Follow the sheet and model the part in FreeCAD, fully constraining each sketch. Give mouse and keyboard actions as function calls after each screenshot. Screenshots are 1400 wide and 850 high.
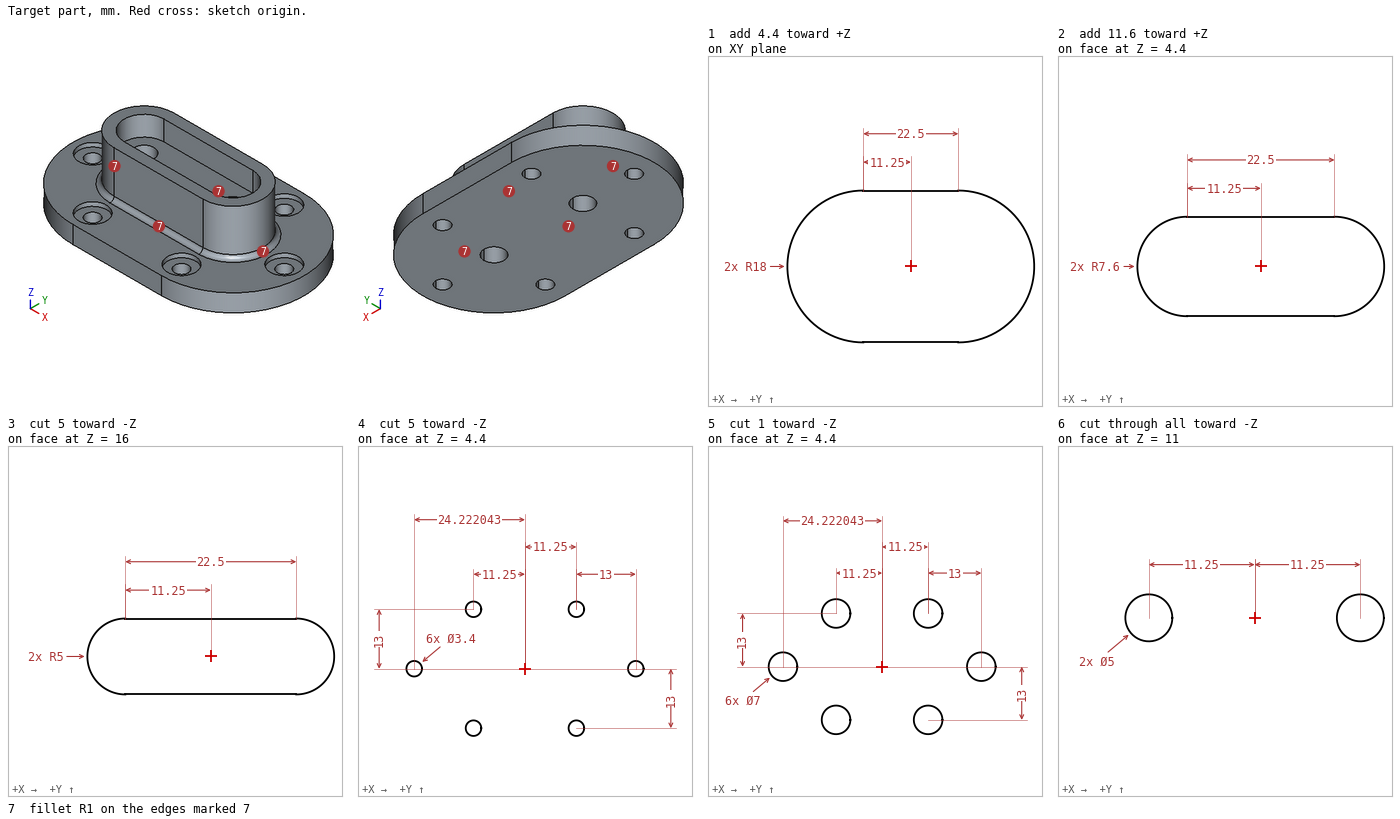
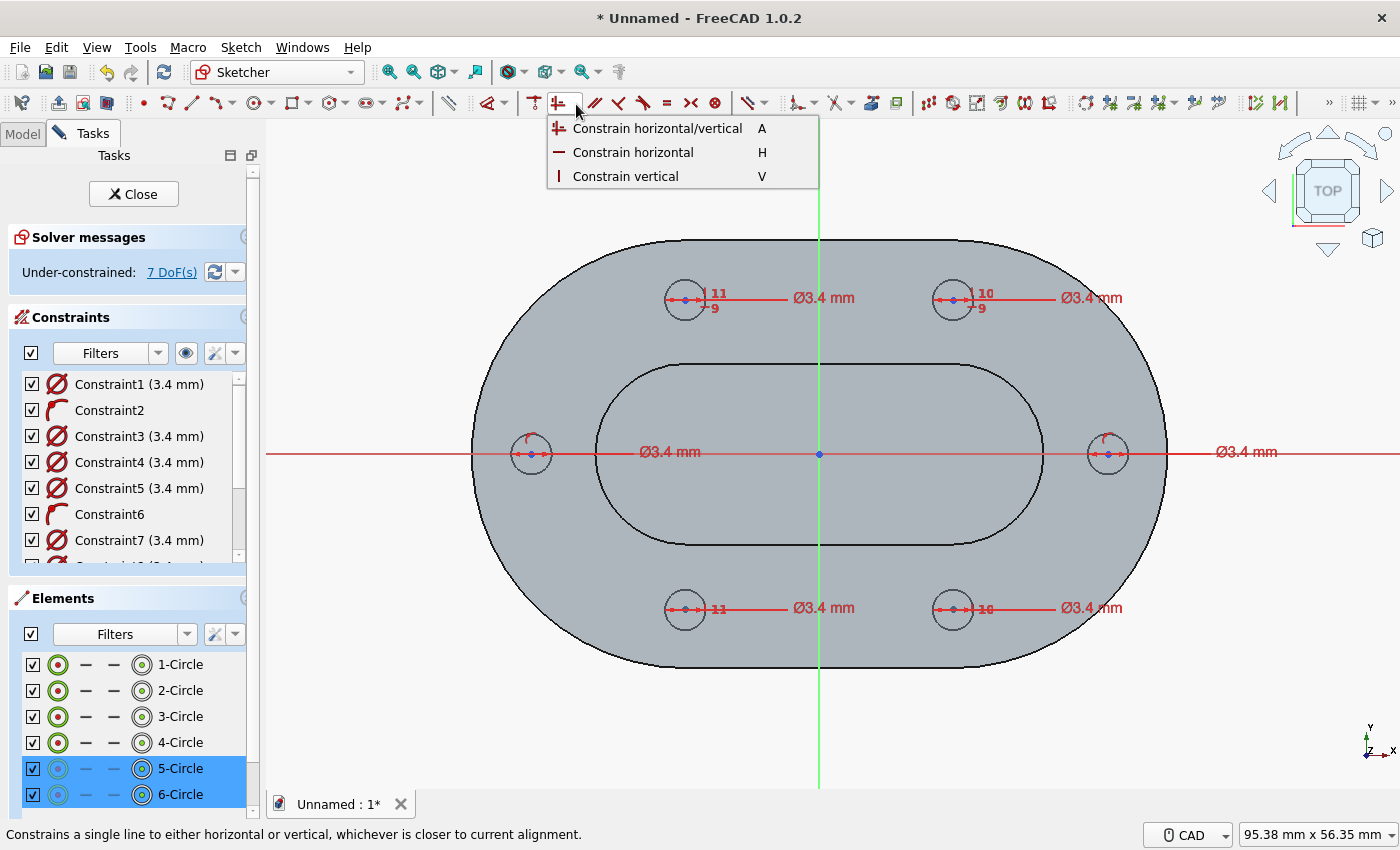
click(683, 152)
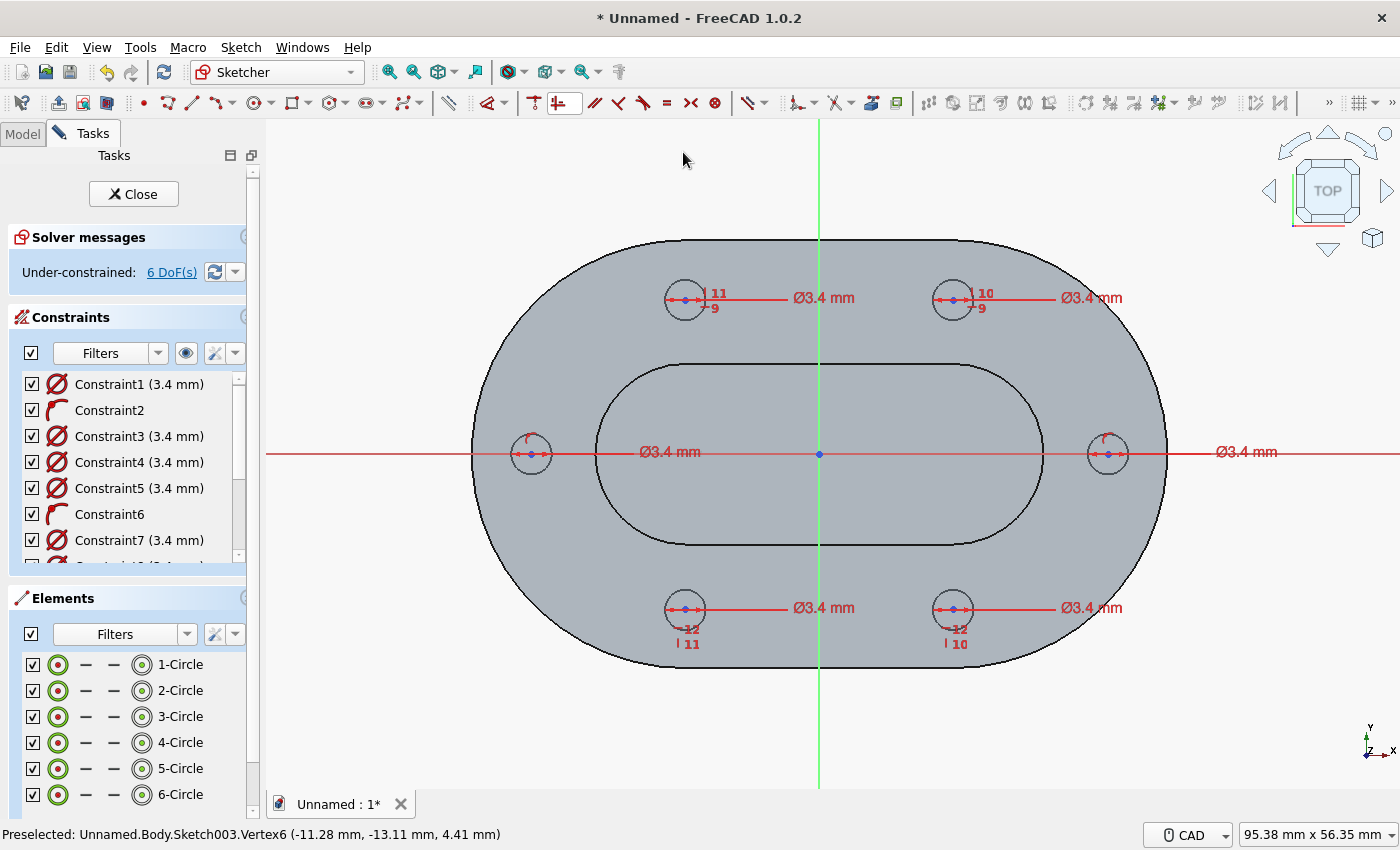
click(488, 104)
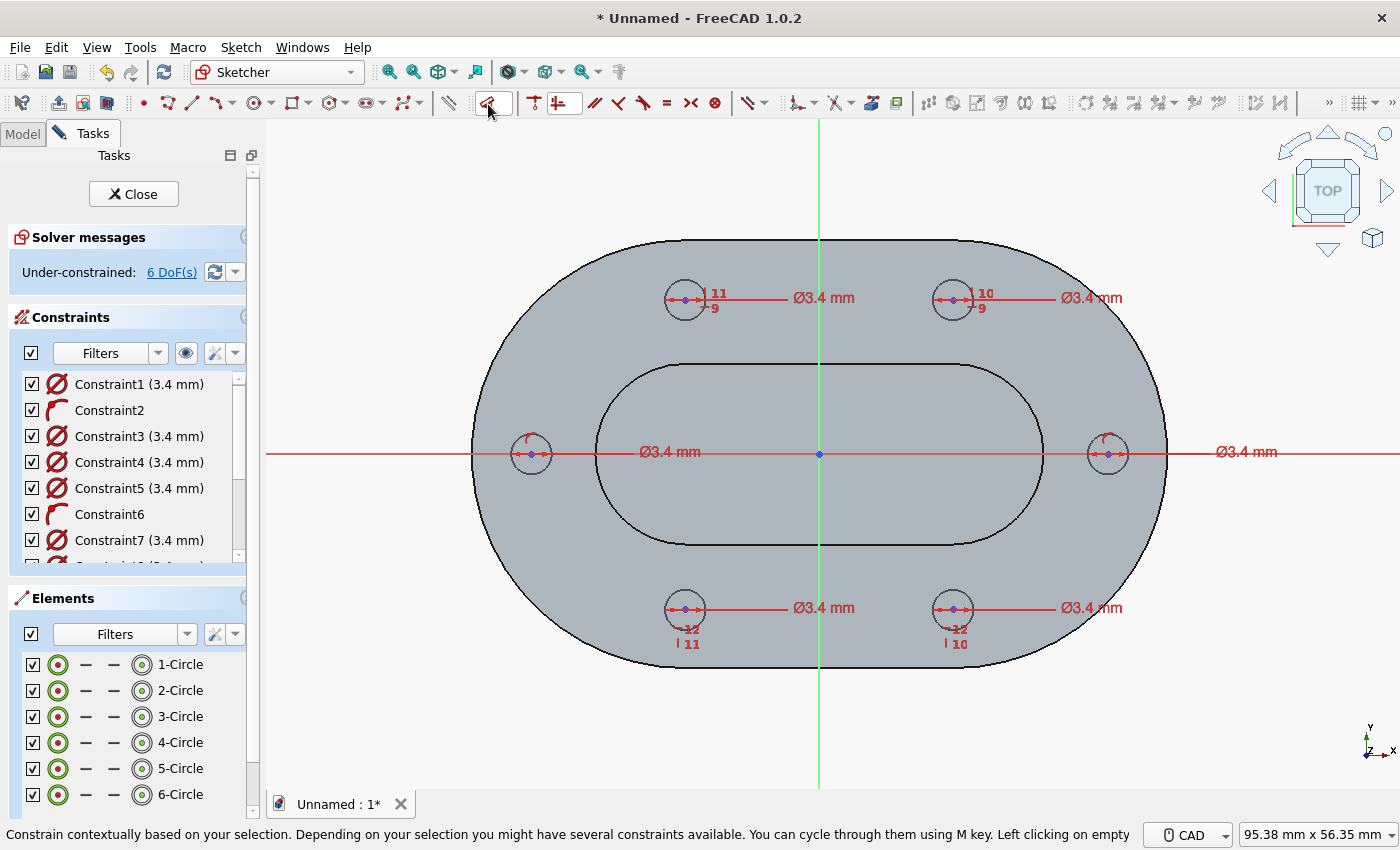
click(685, 300)
click(651, 377)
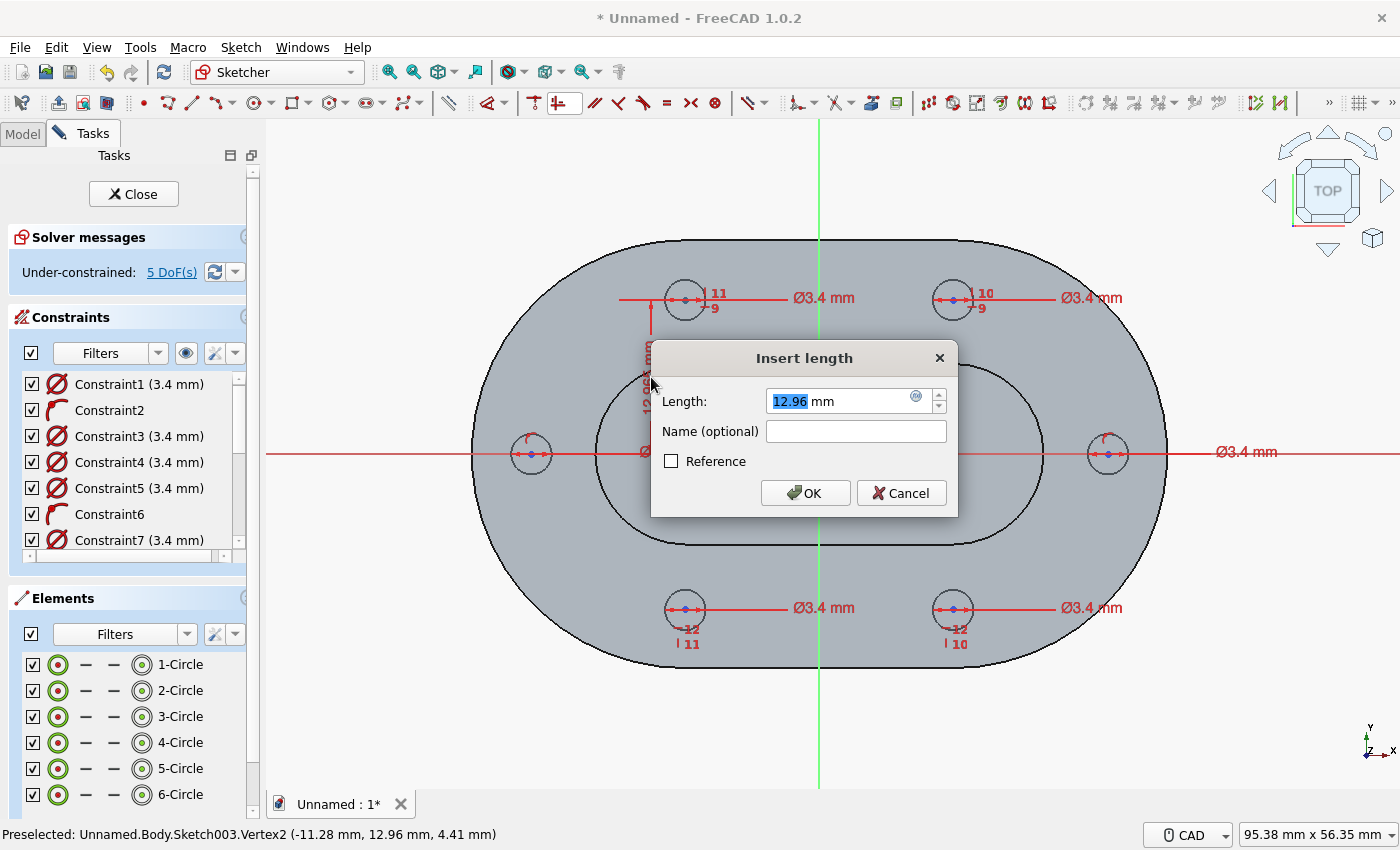
text(13)
key(Return)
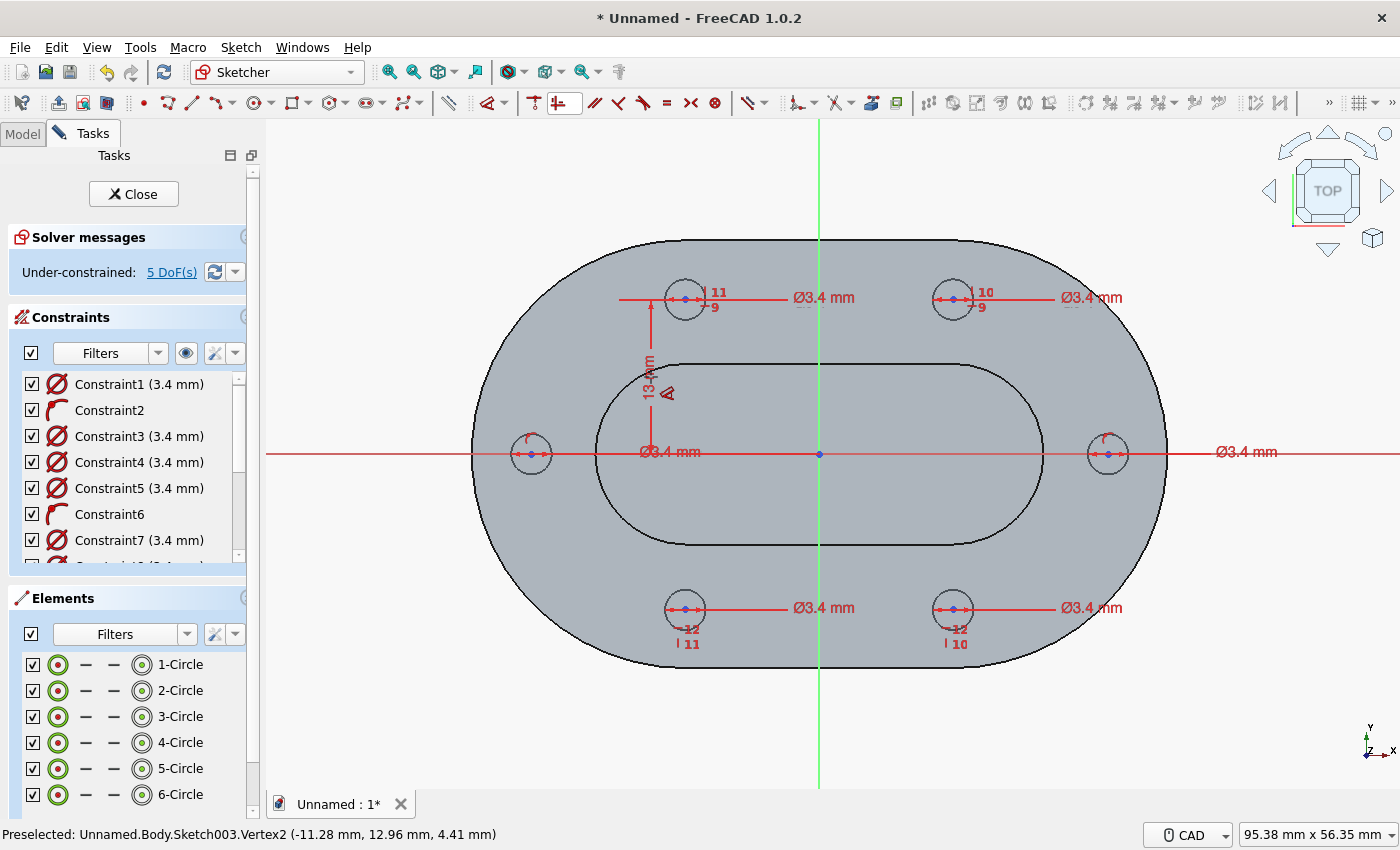
click(953, 610)
click(987, 532)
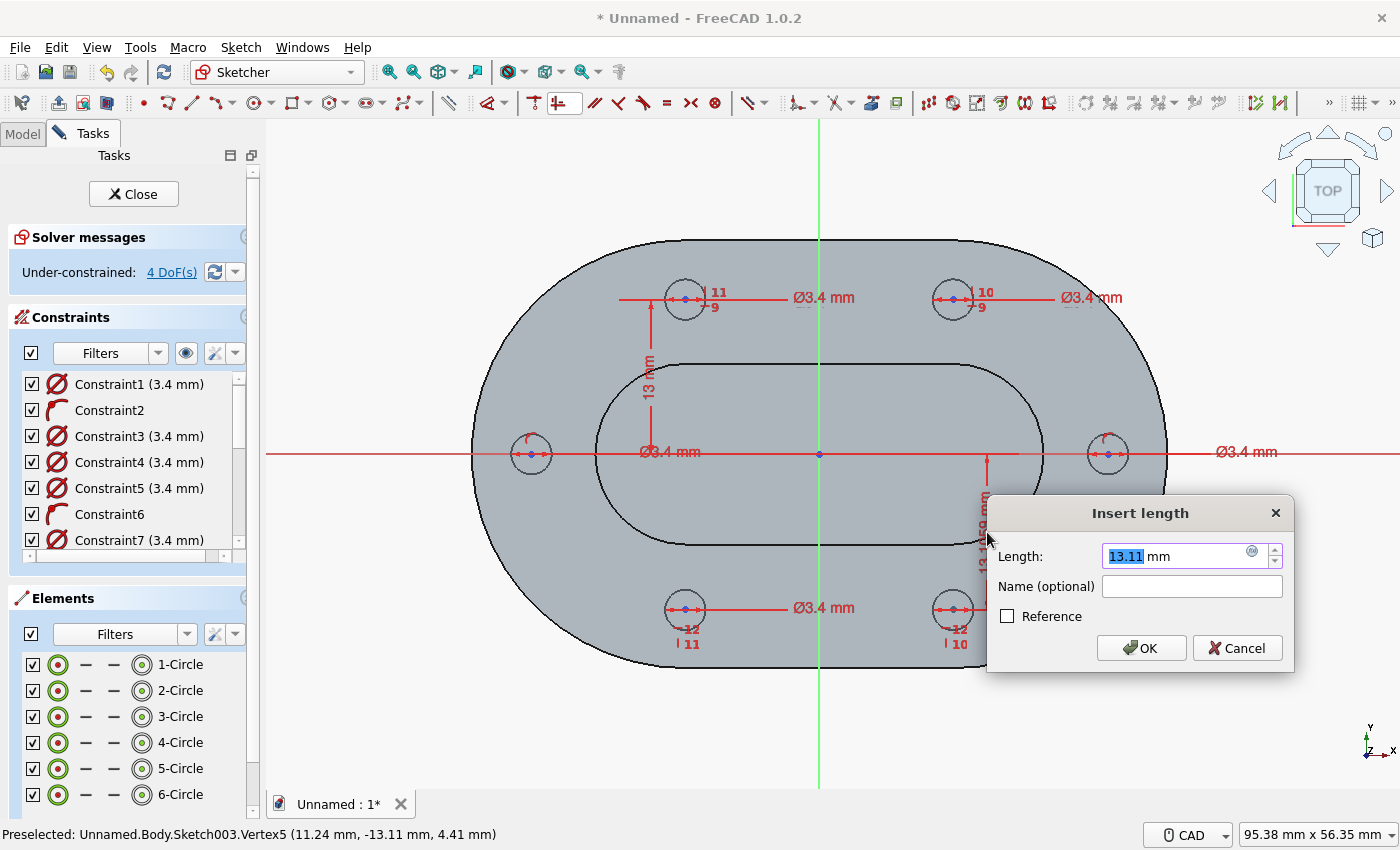
text(13)
key(Return)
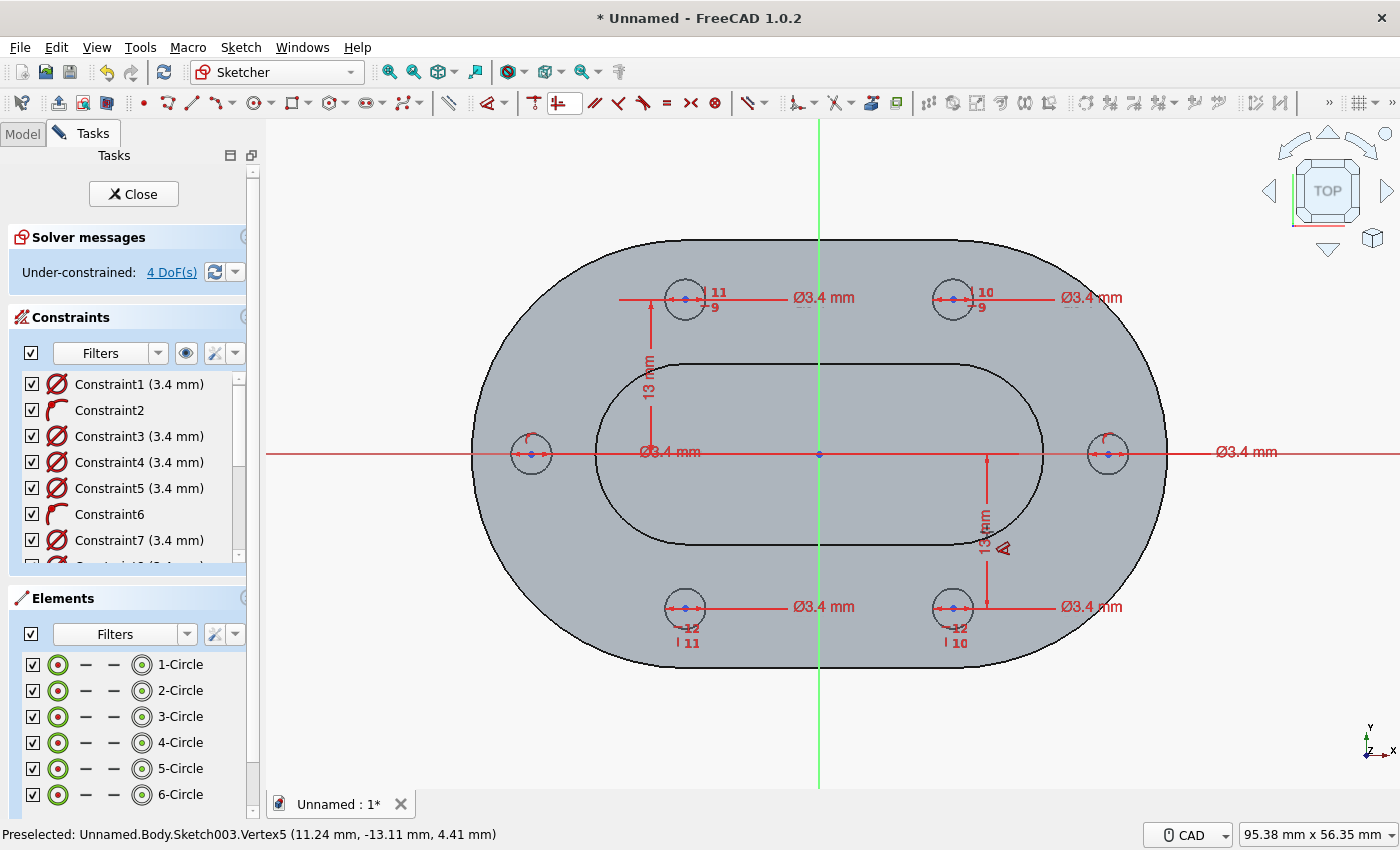
click(953, 300)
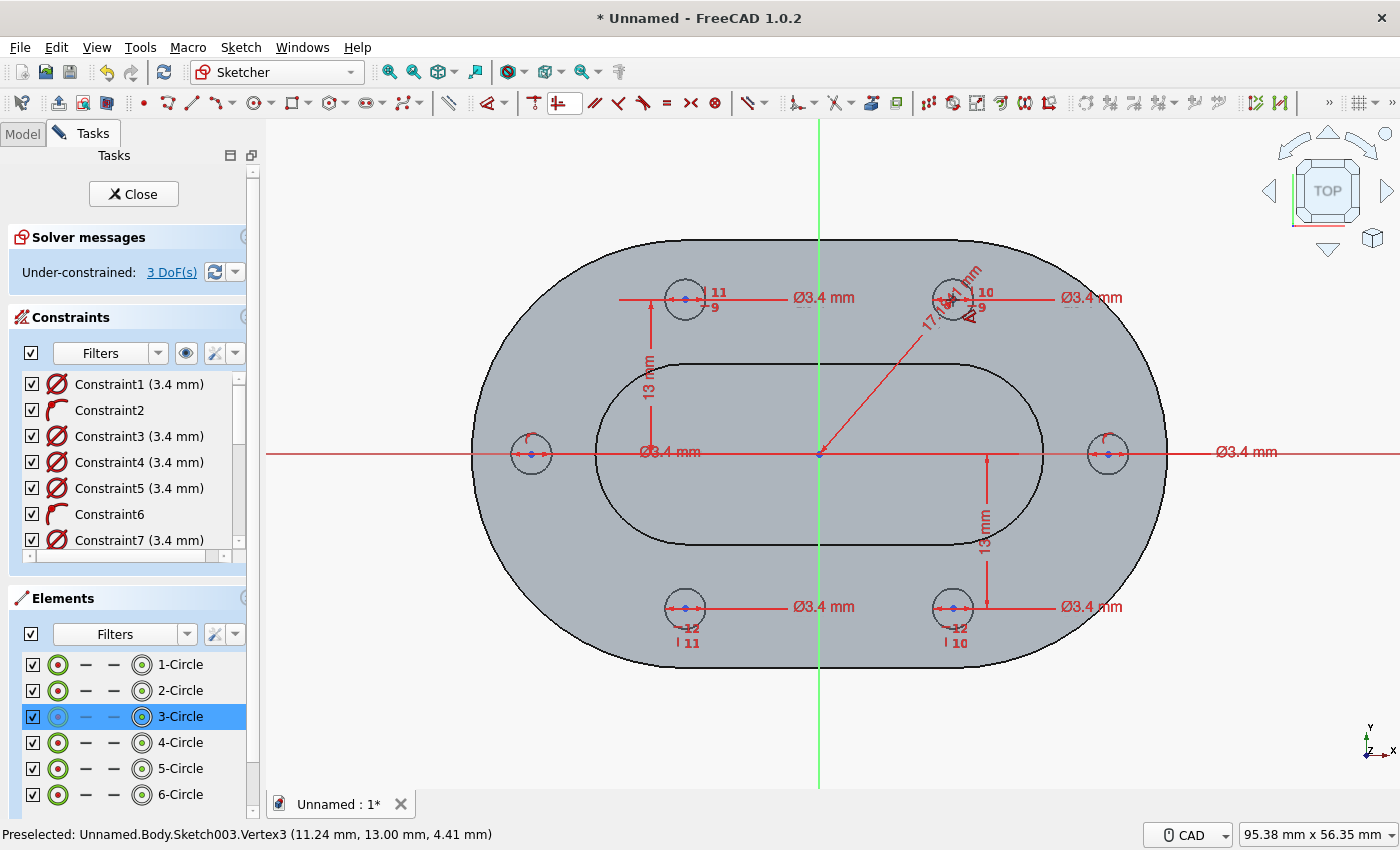
click(1108, 454)
click(1031, 266)